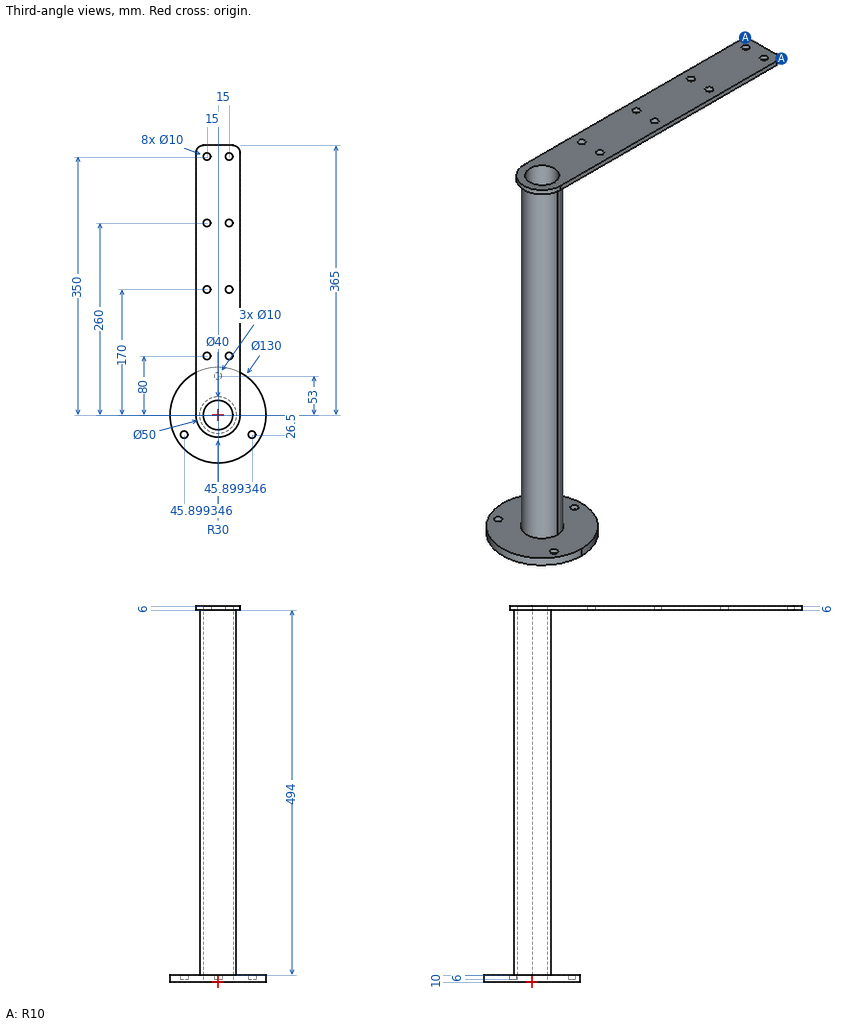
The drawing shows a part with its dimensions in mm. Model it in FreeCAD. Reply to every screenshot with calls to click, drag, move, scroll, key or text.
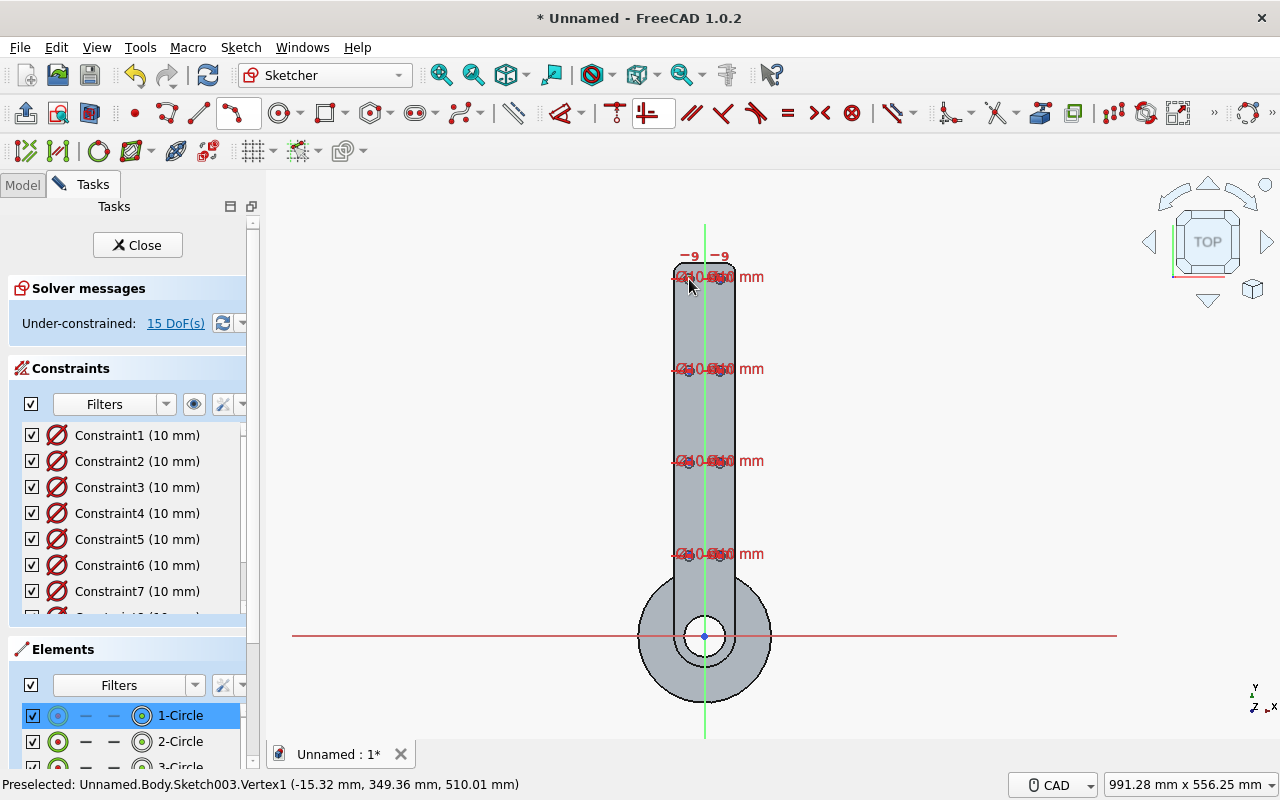
click(689, 371)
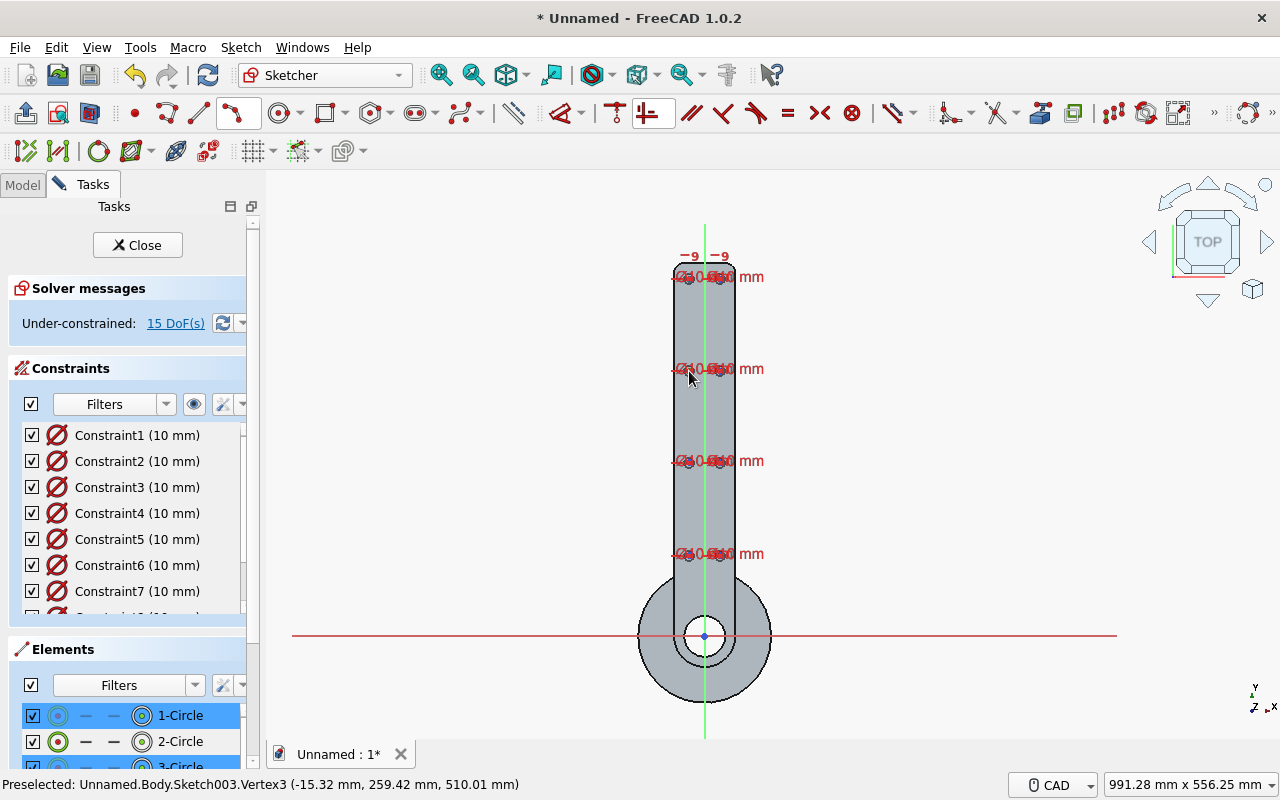
click(670, 114)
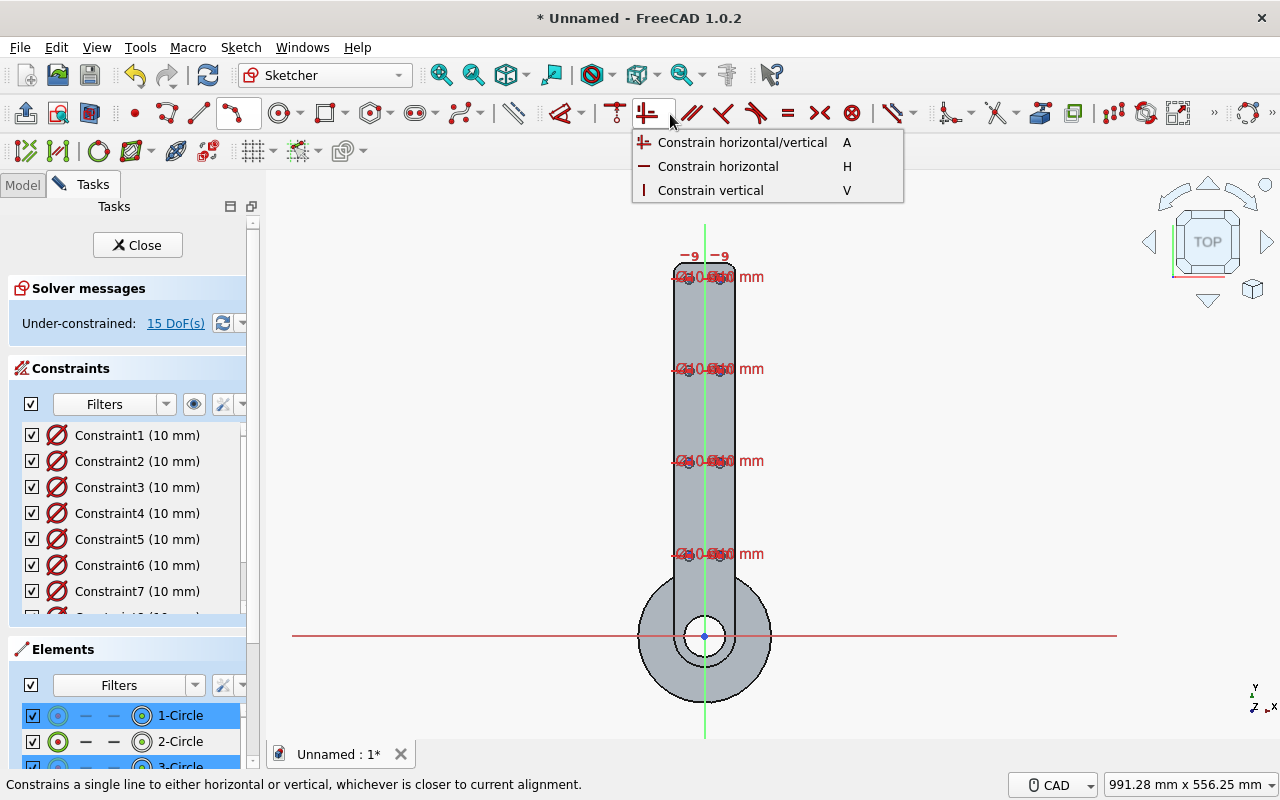
click(768, 190)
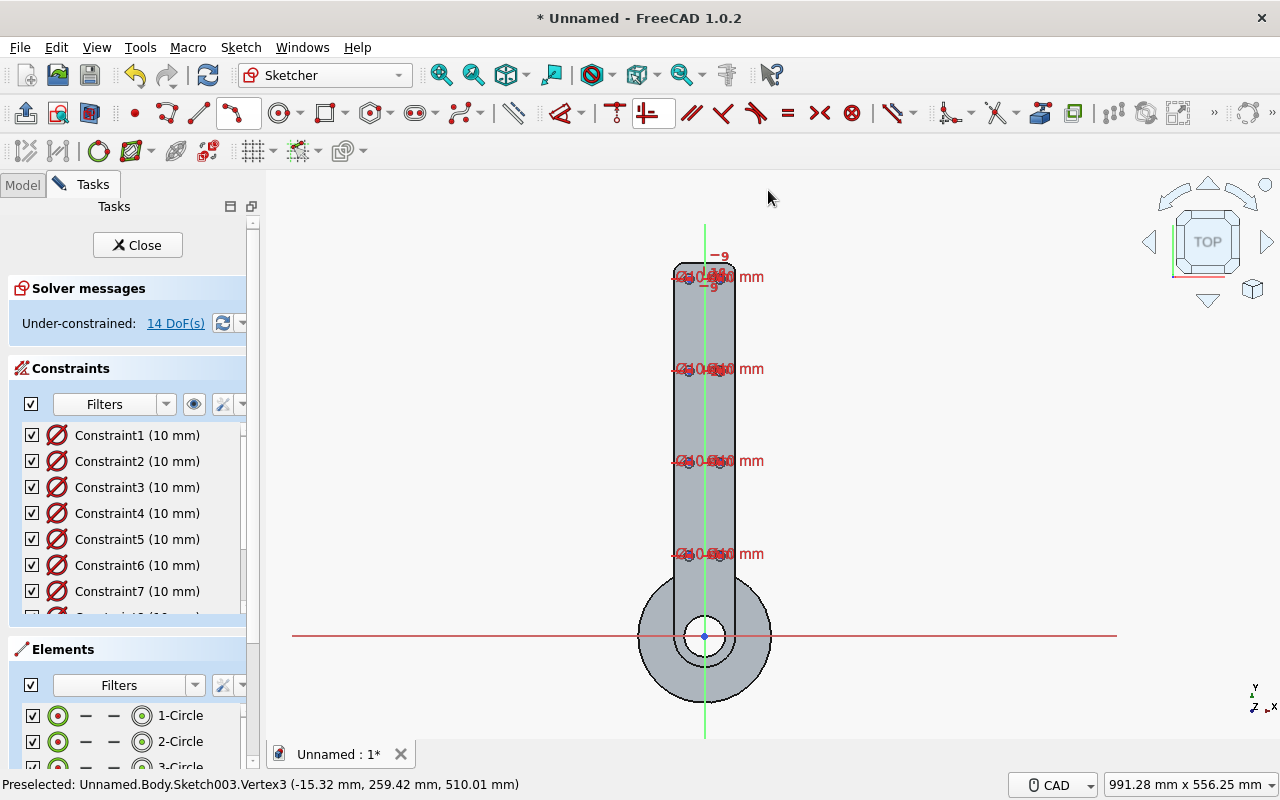
click(720, 279)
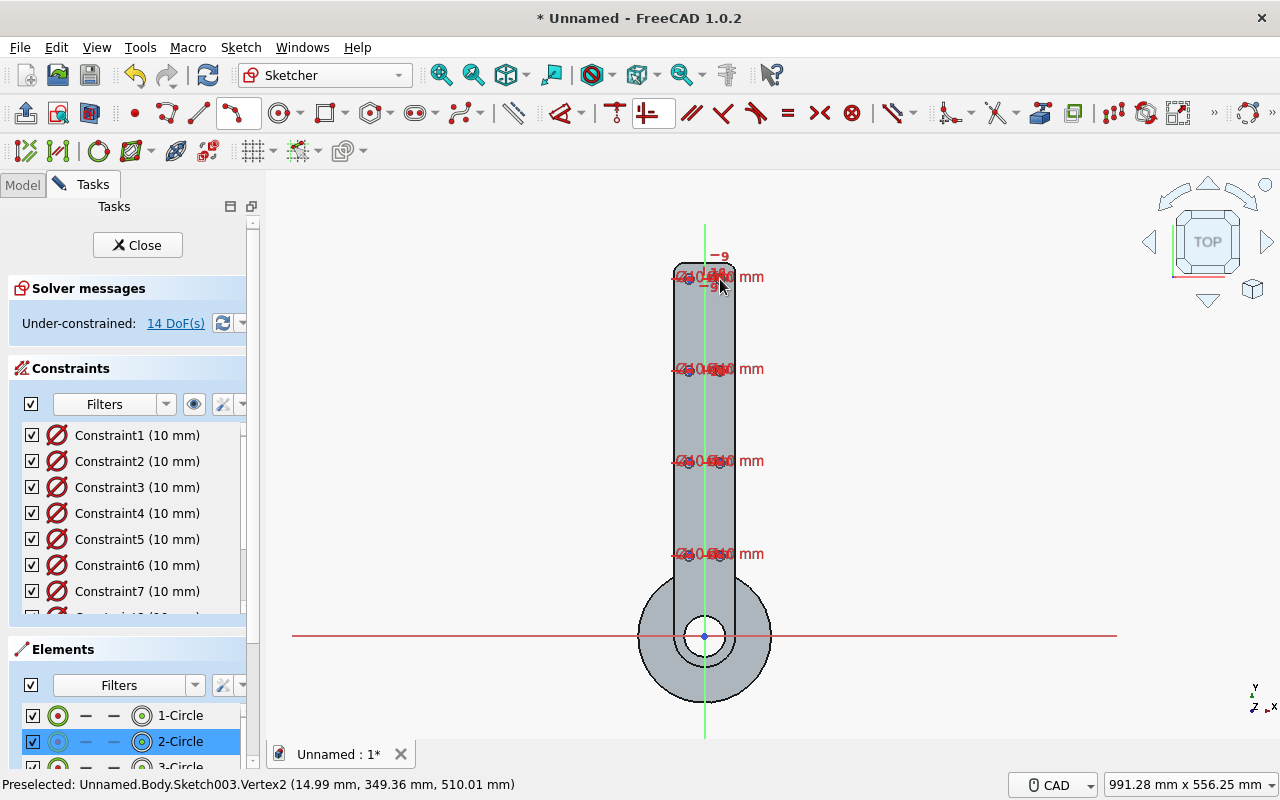
scroll(720, 371, up, 4)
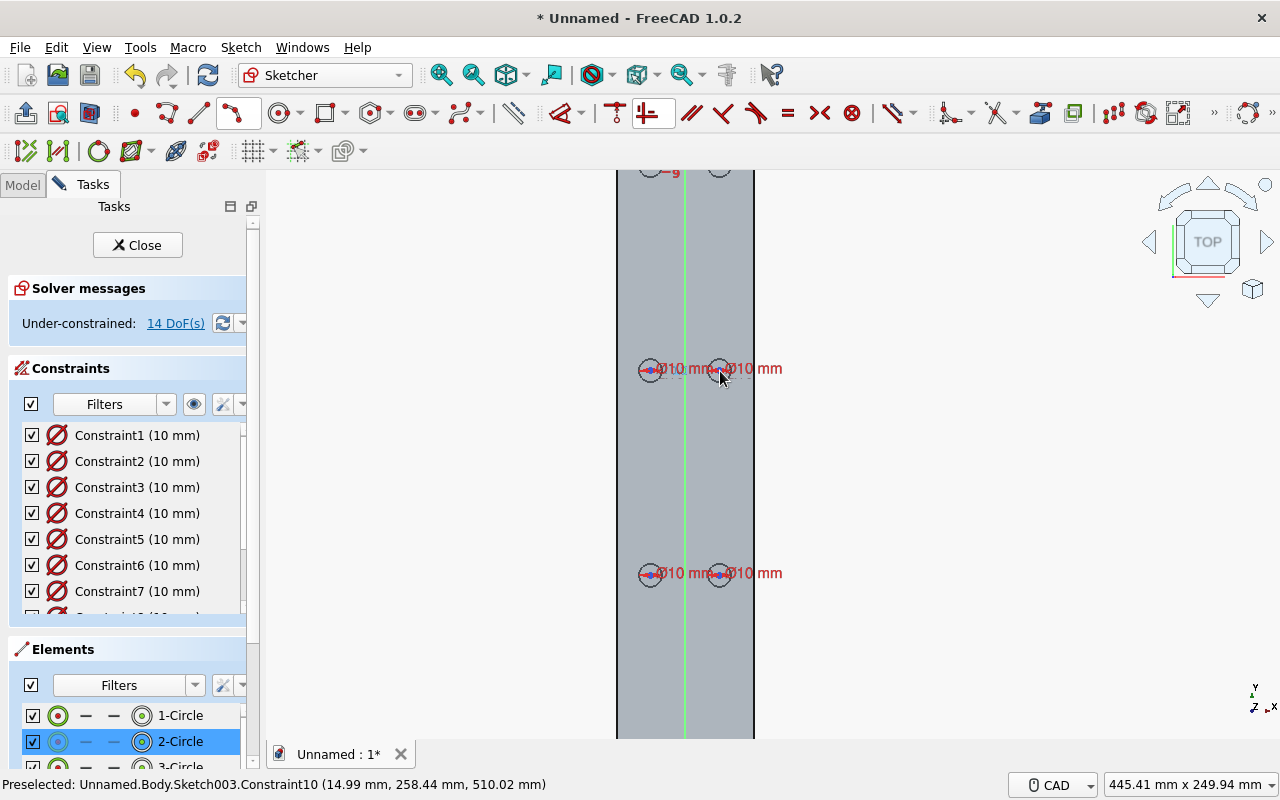
click(719, 371)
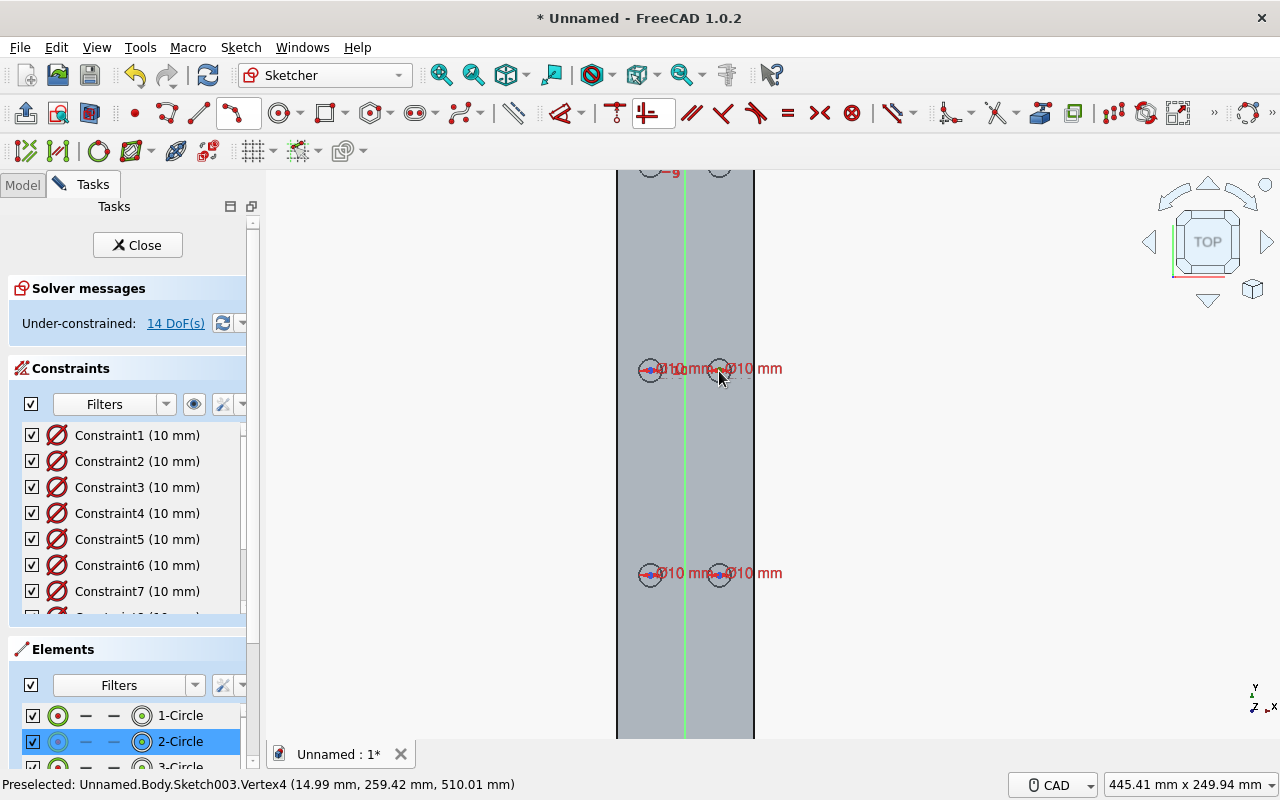
click(670, 114)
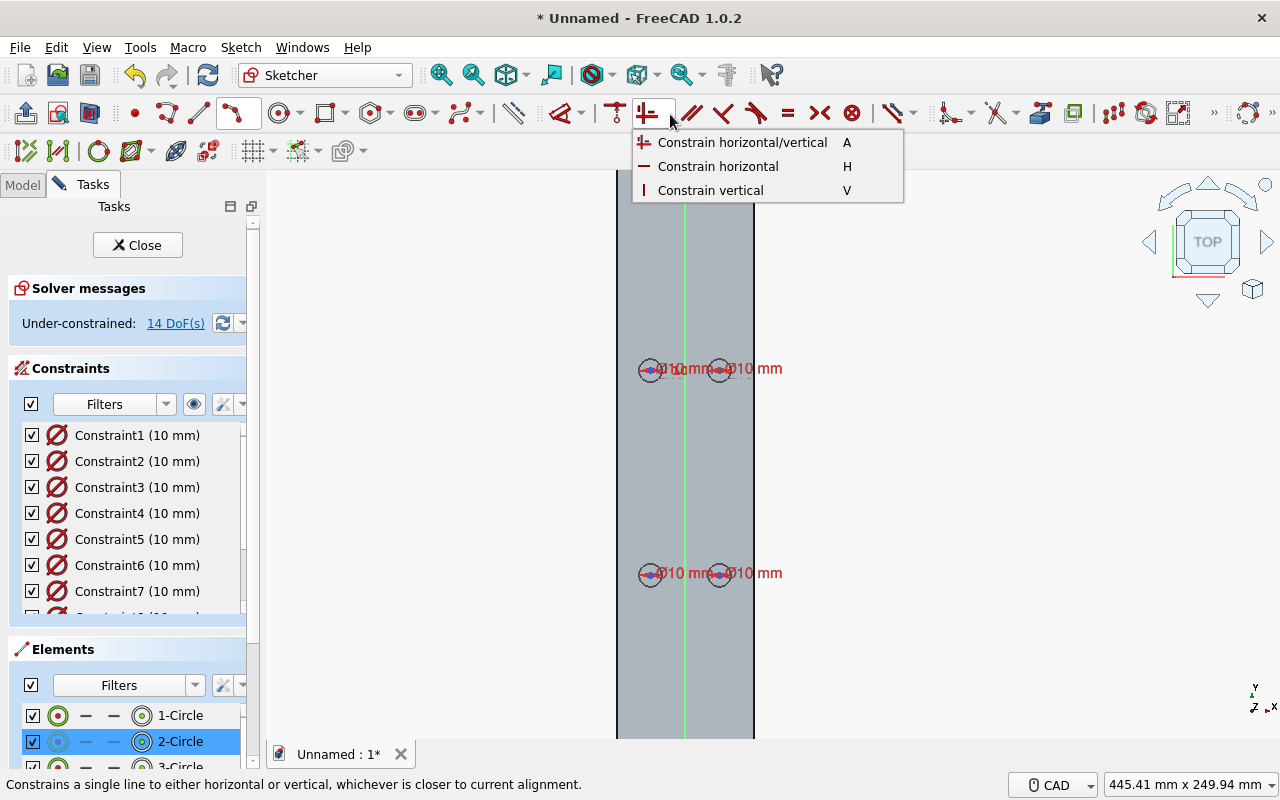
click(768, 190)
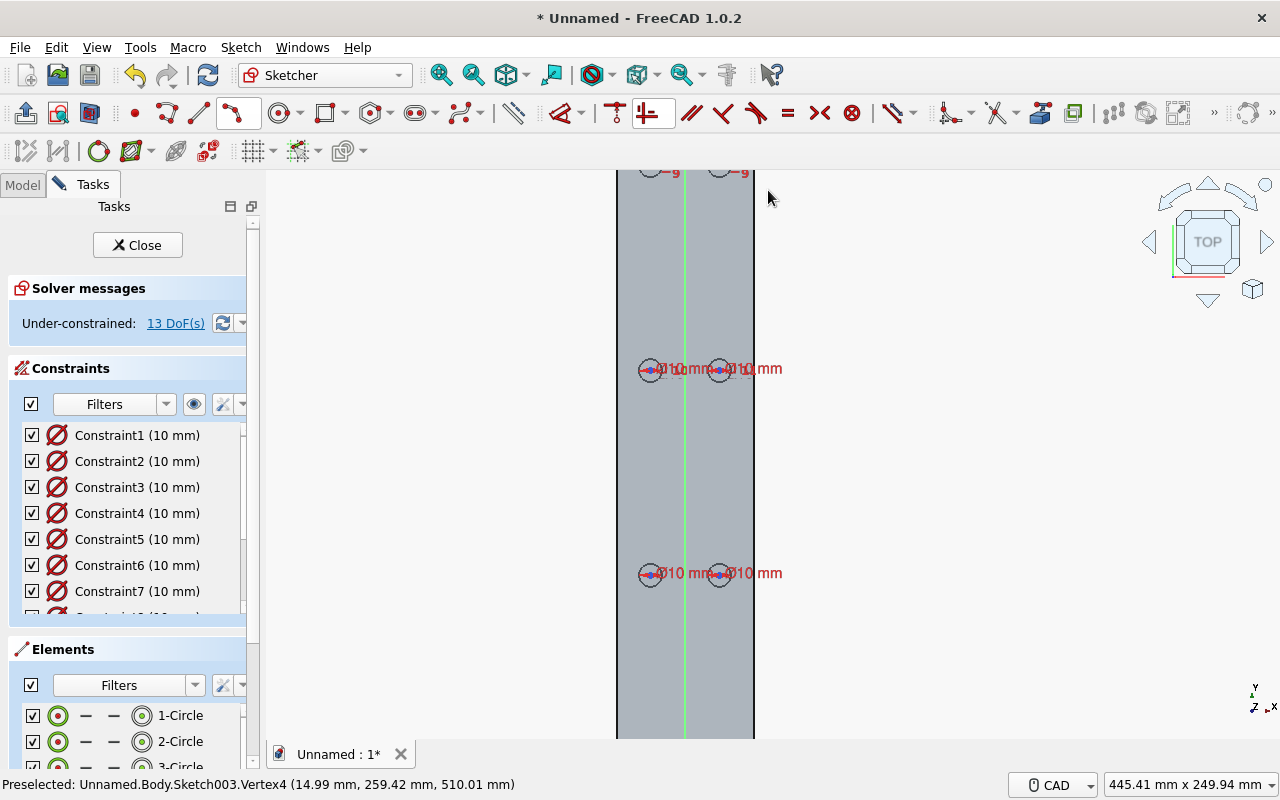
click(650, 371)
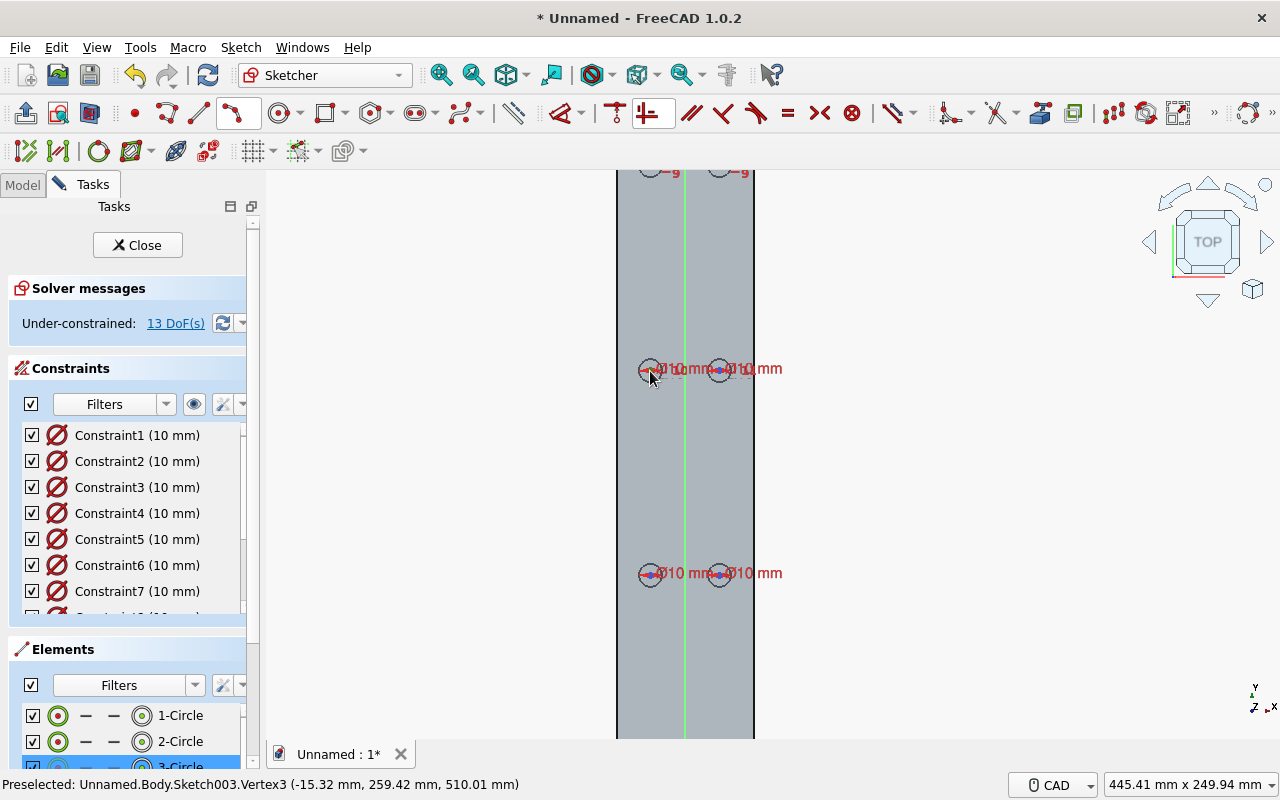
click(719, 371)